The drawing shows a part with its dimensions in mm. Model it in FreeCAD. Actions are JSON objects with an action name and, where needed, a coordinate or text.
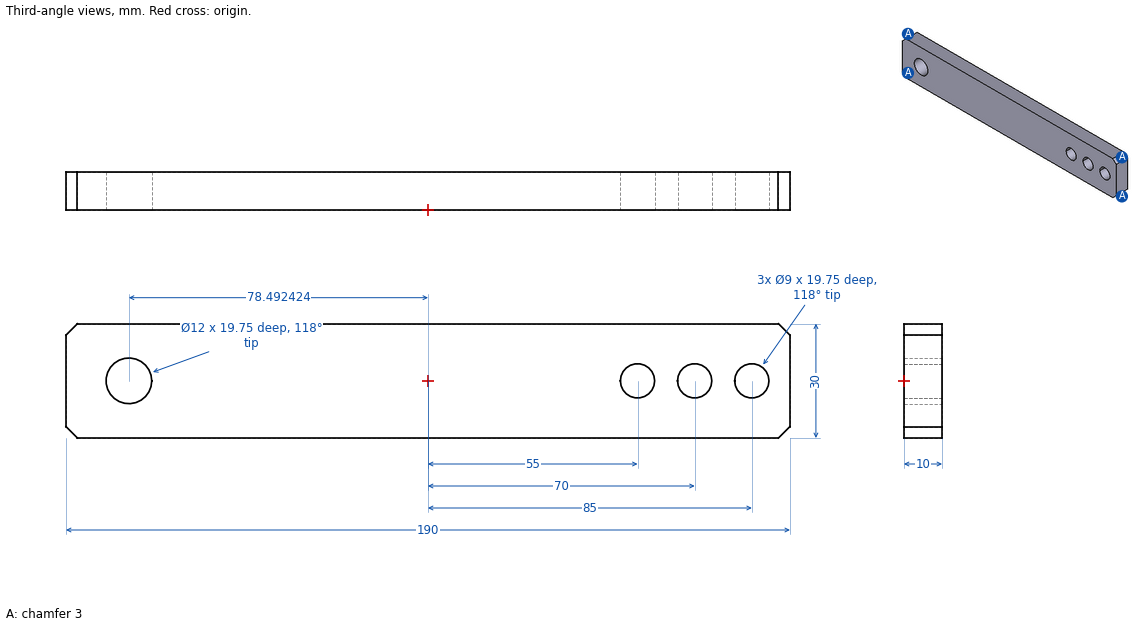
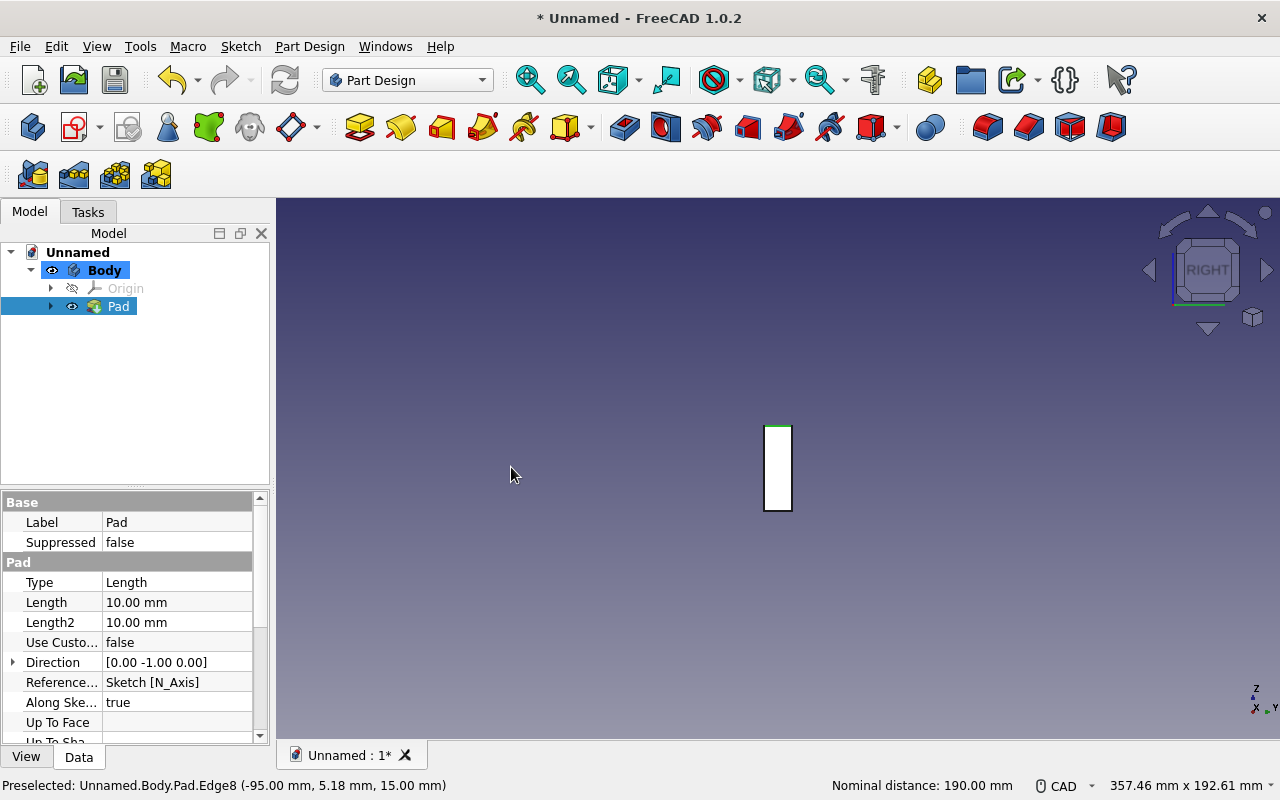
{"action": "key", "text": "v f"}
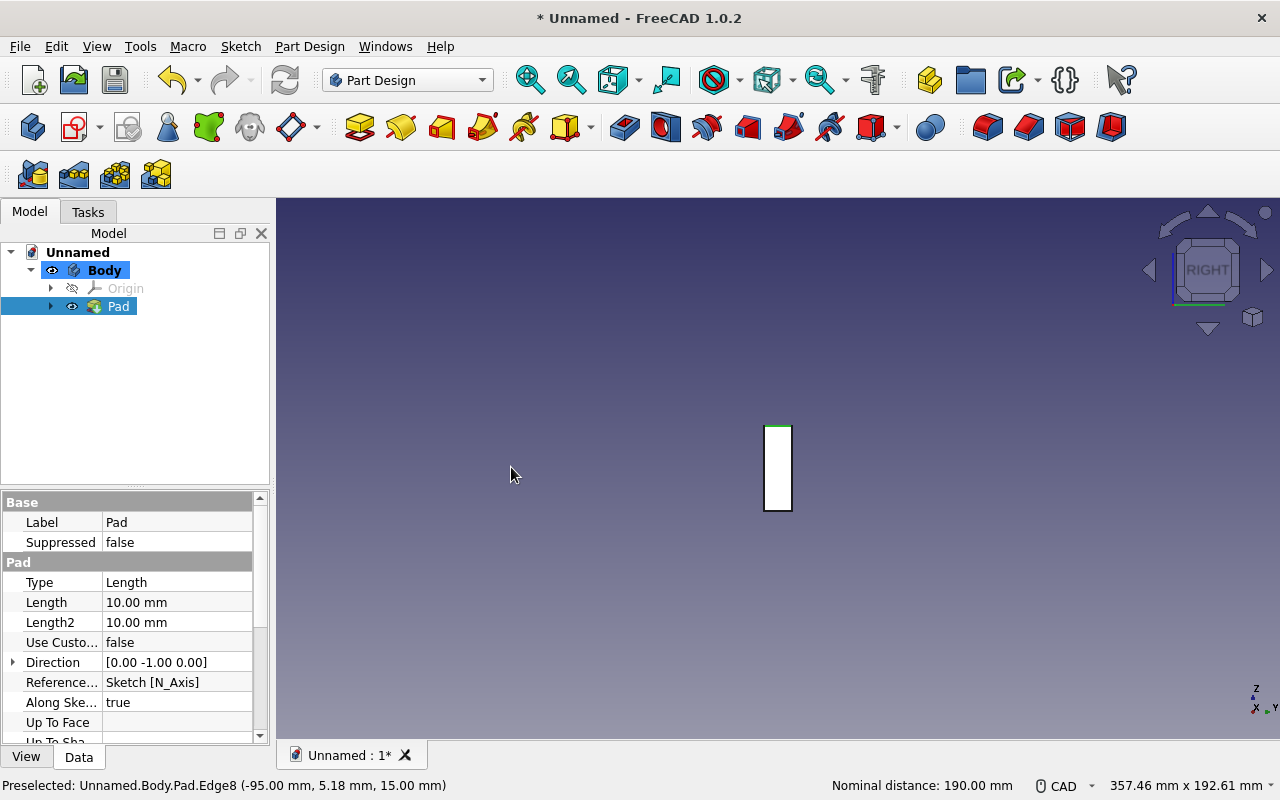
{"action": "left_click", "coordinate": [778, 510], "text": "ctrl"}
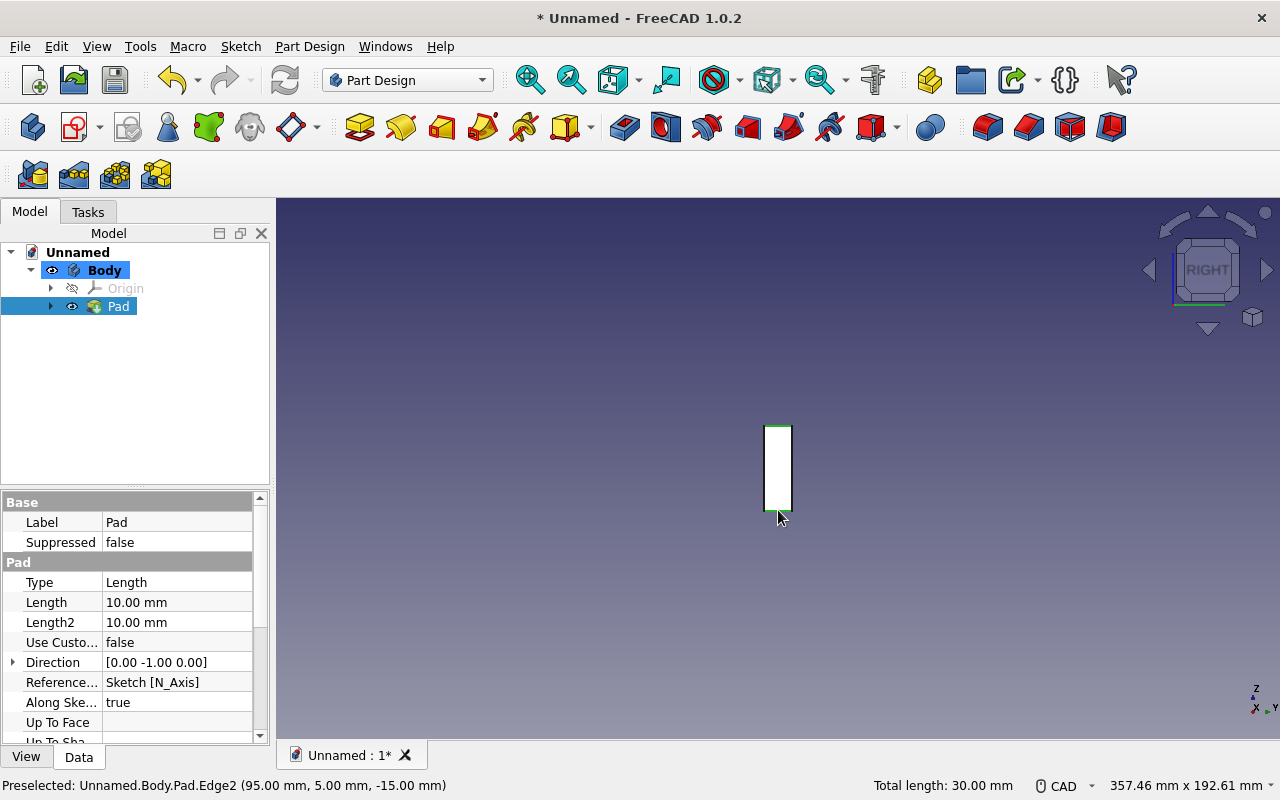
{"action": "key", "text": "5"}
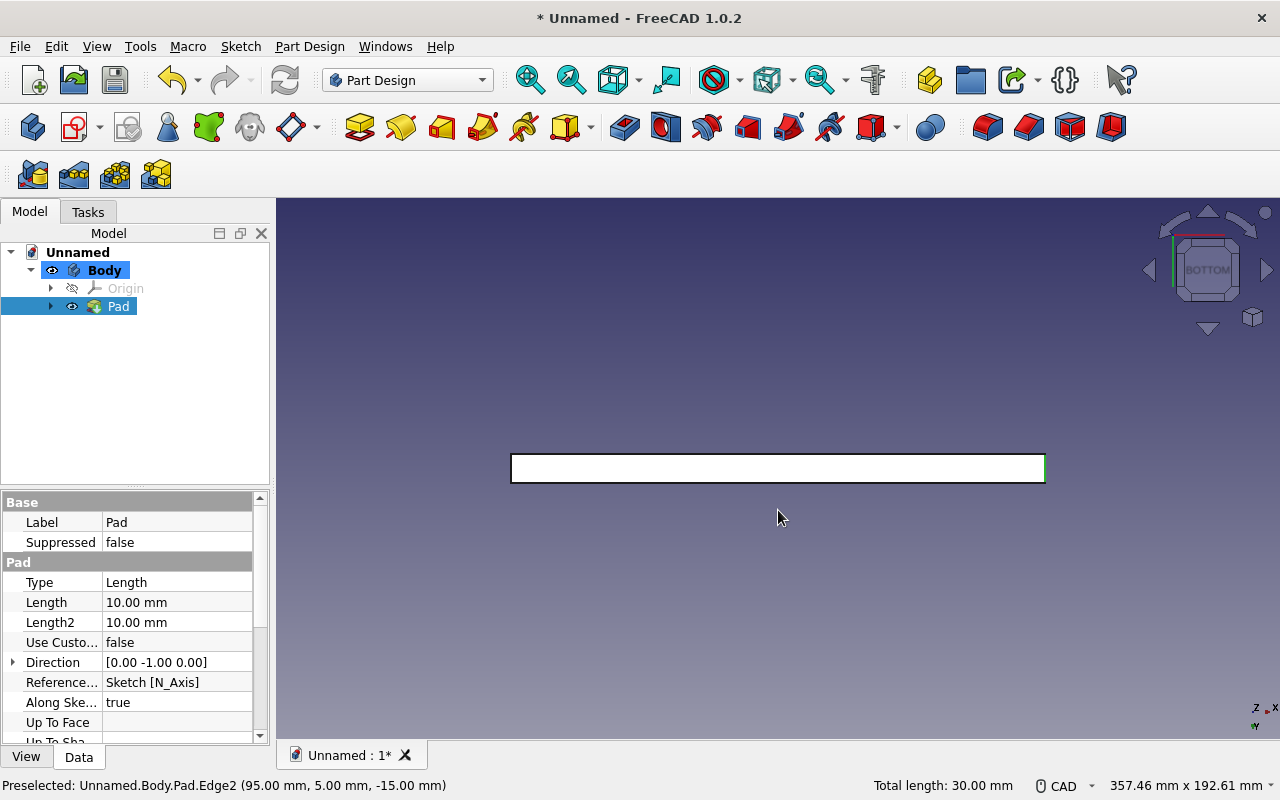
{"action": "left_click", "coordinate": [511, 467], "text": "ctrl"}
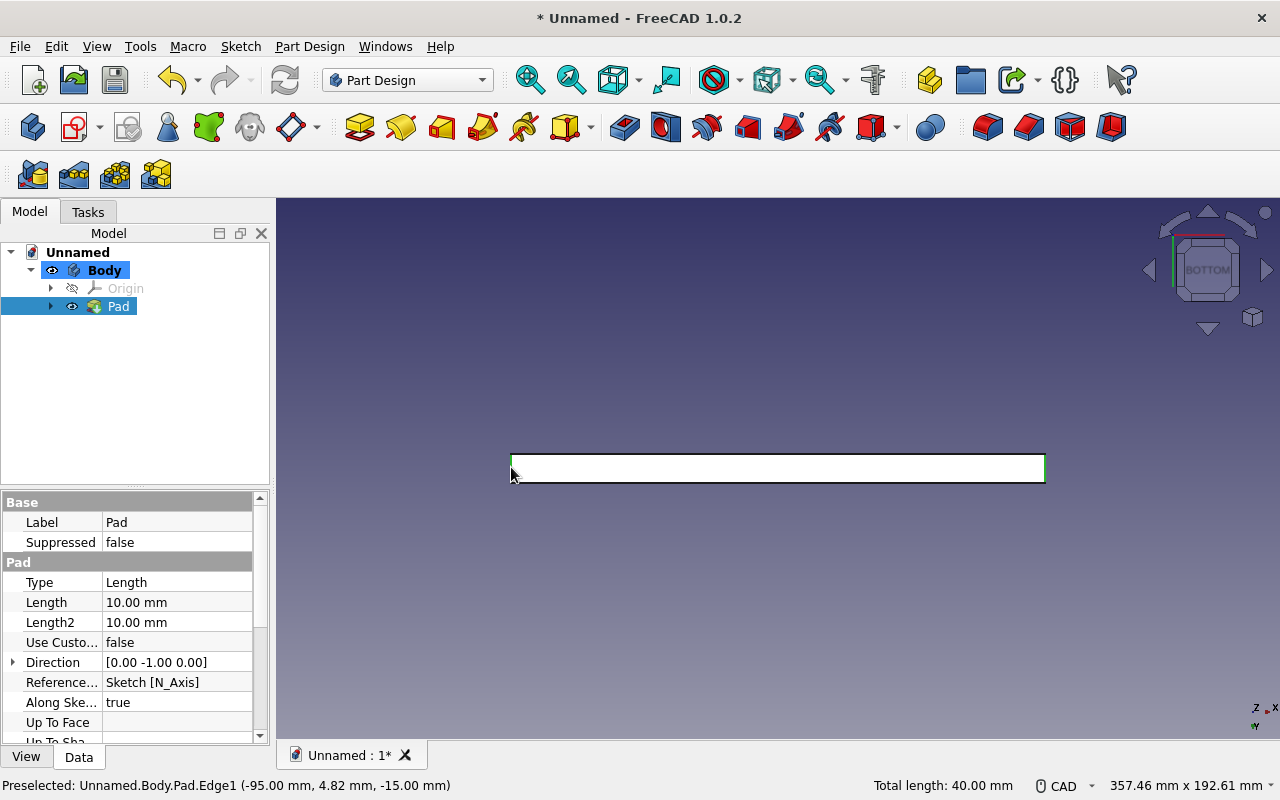
{"action": "left_click", "coordinate": [1029, 128]}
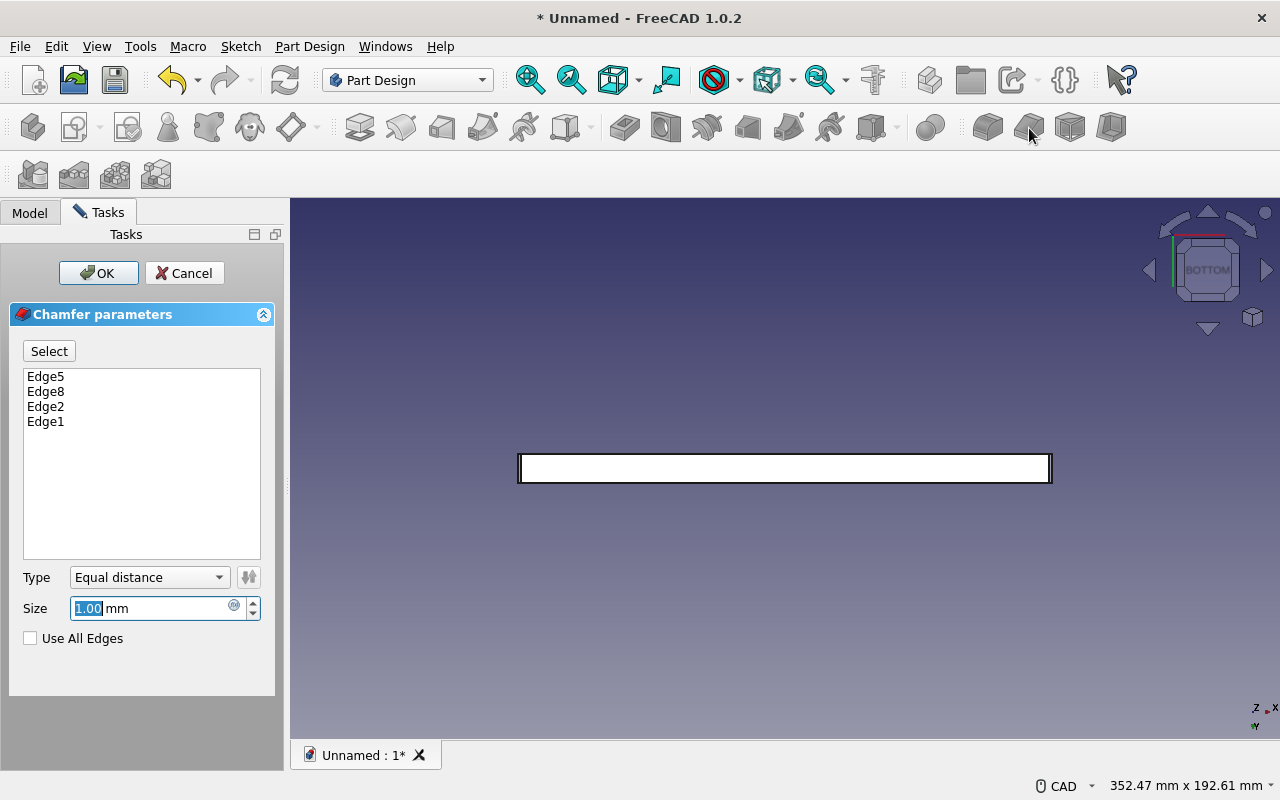
{"action": "type", "text": "3"}
{"action": "key", "text": "Tab"}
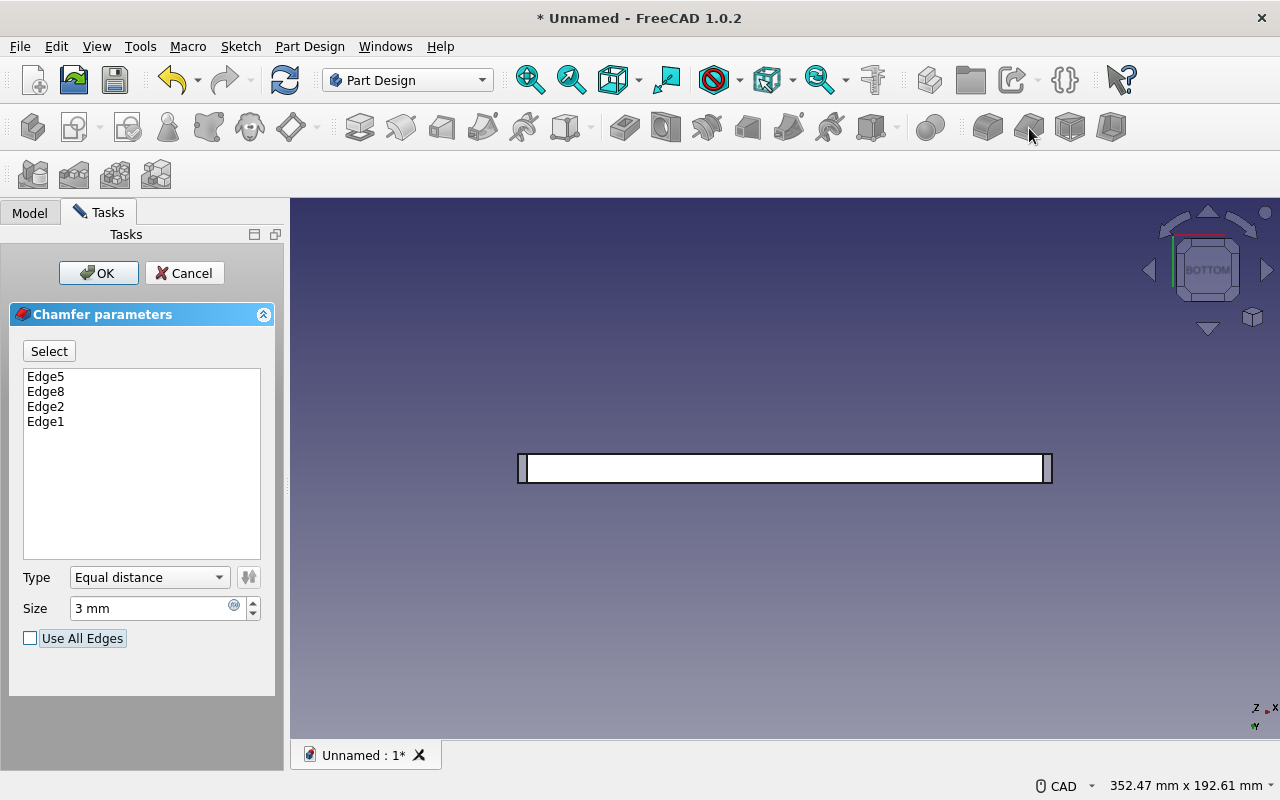
{"action": "left_click", "coordinate": [99, 273]}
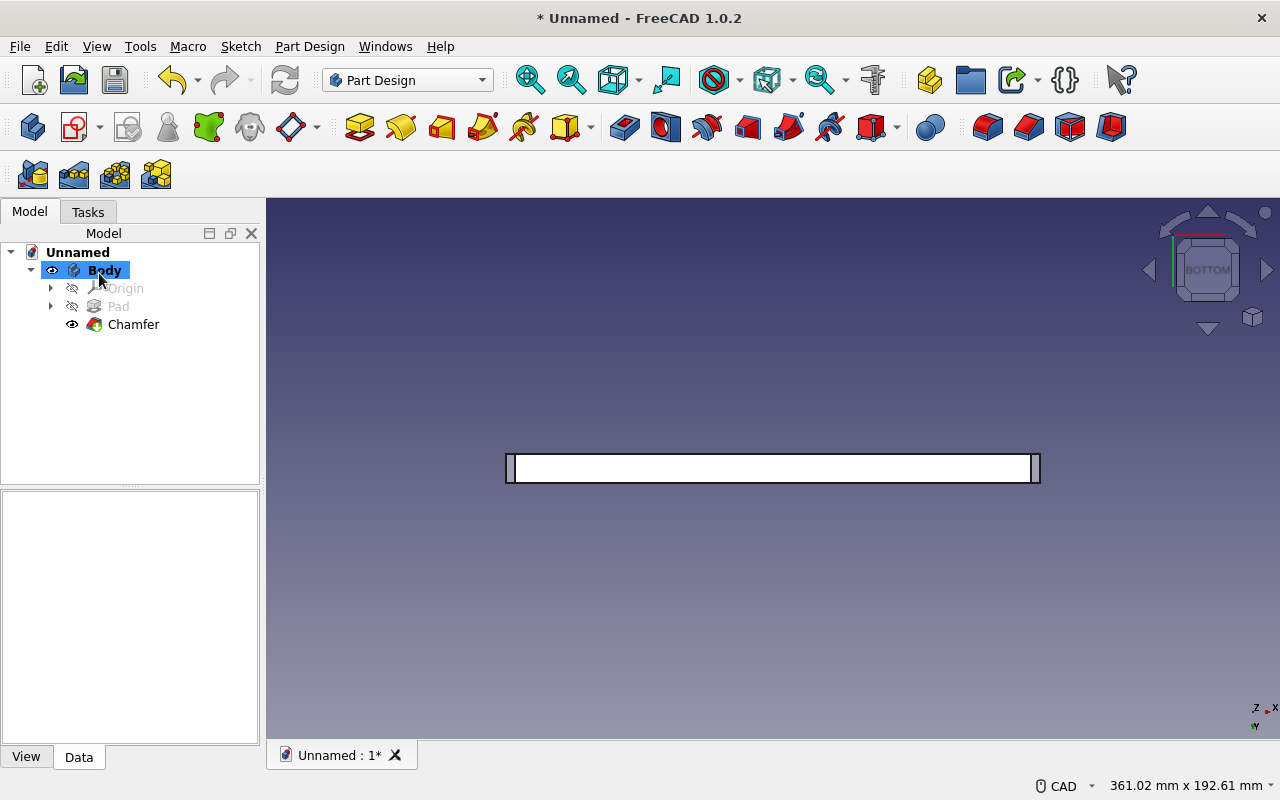
{"action": "key", "text": "4"}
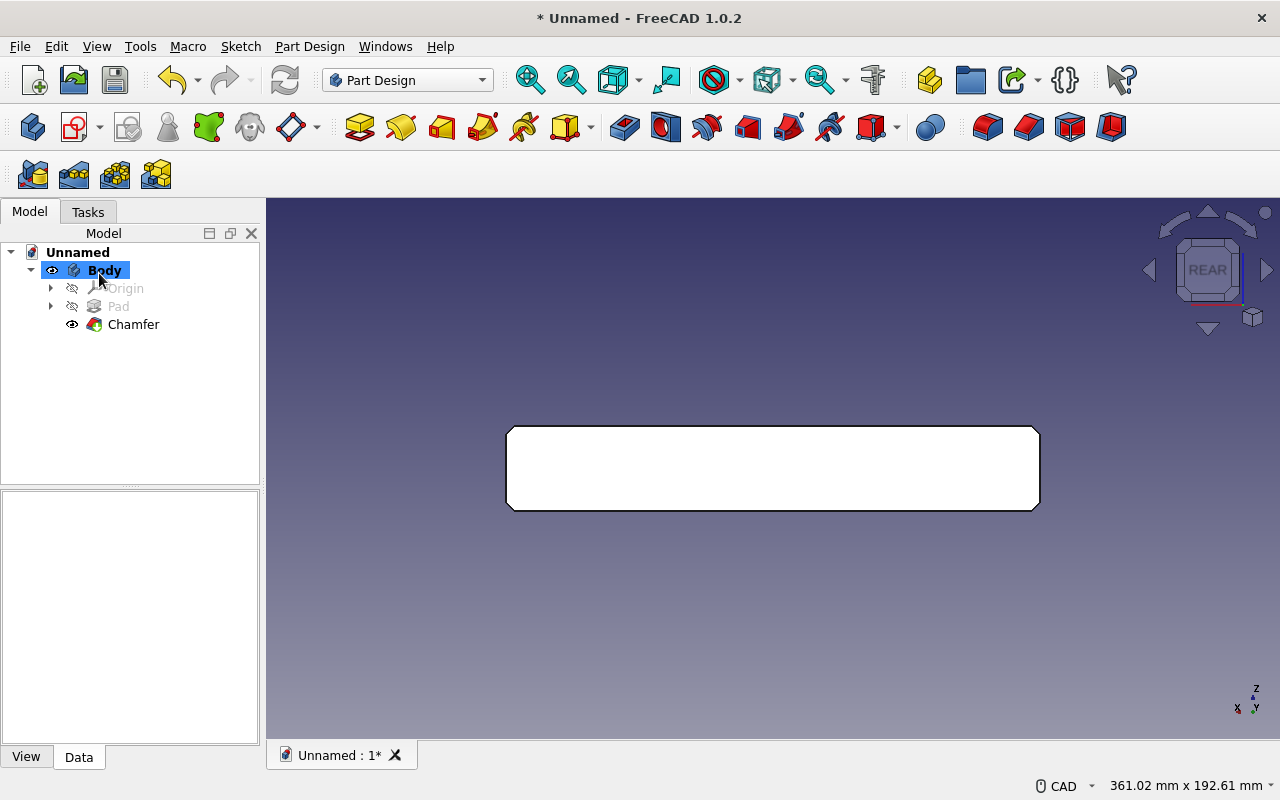
{"action": "left_click", "coordinate": [621, 468]}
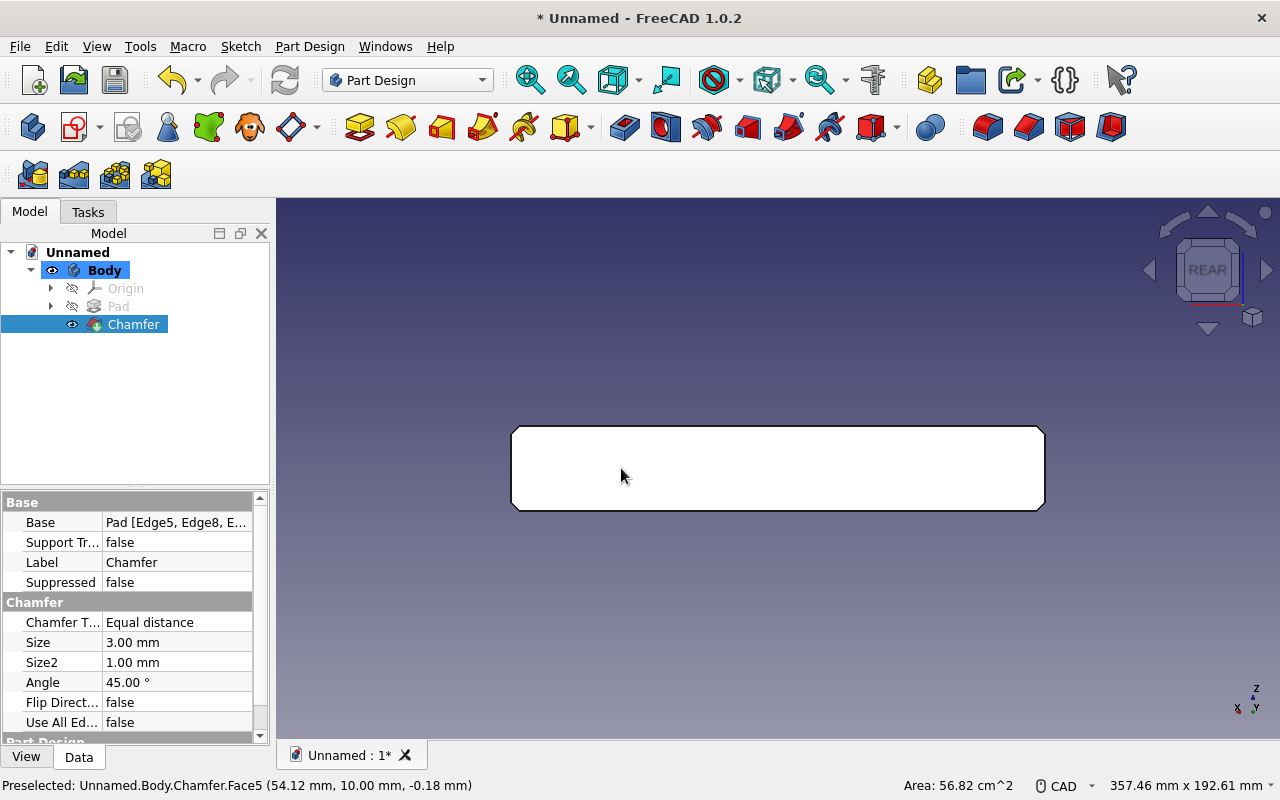
{"action": "left_click", "coordinate": [74, 128]}